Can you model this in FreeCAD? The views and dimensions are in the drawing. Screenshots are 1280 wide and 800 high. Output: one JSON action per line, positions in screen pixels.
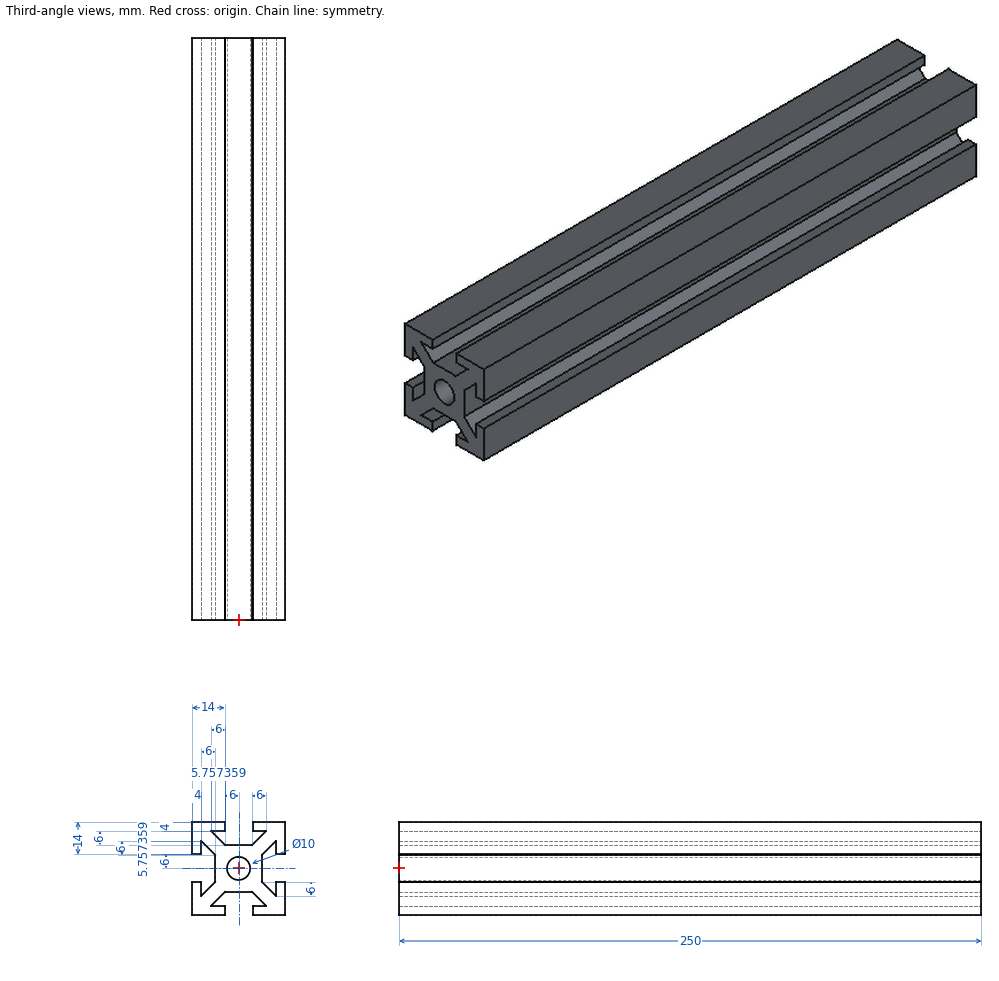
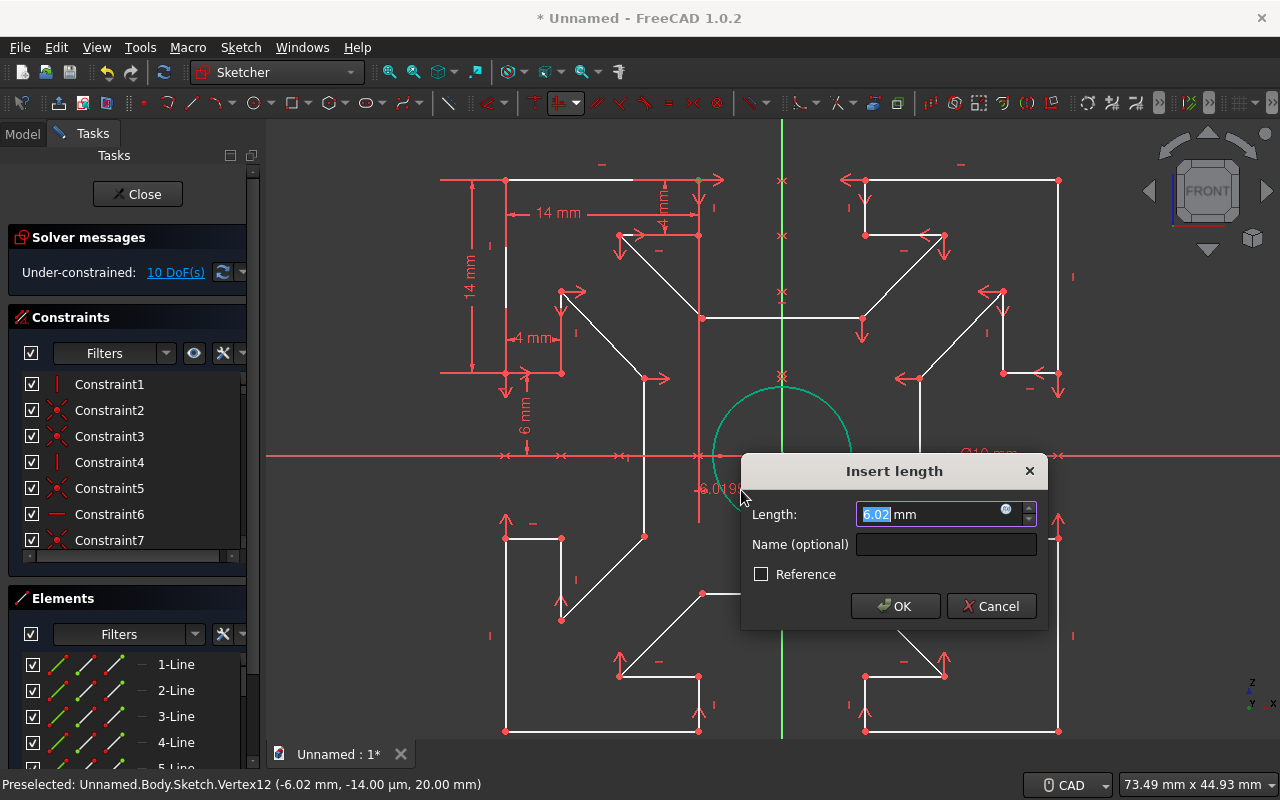
{"action": "type", "text": "6"}
{"action": "key", "text": "Return"}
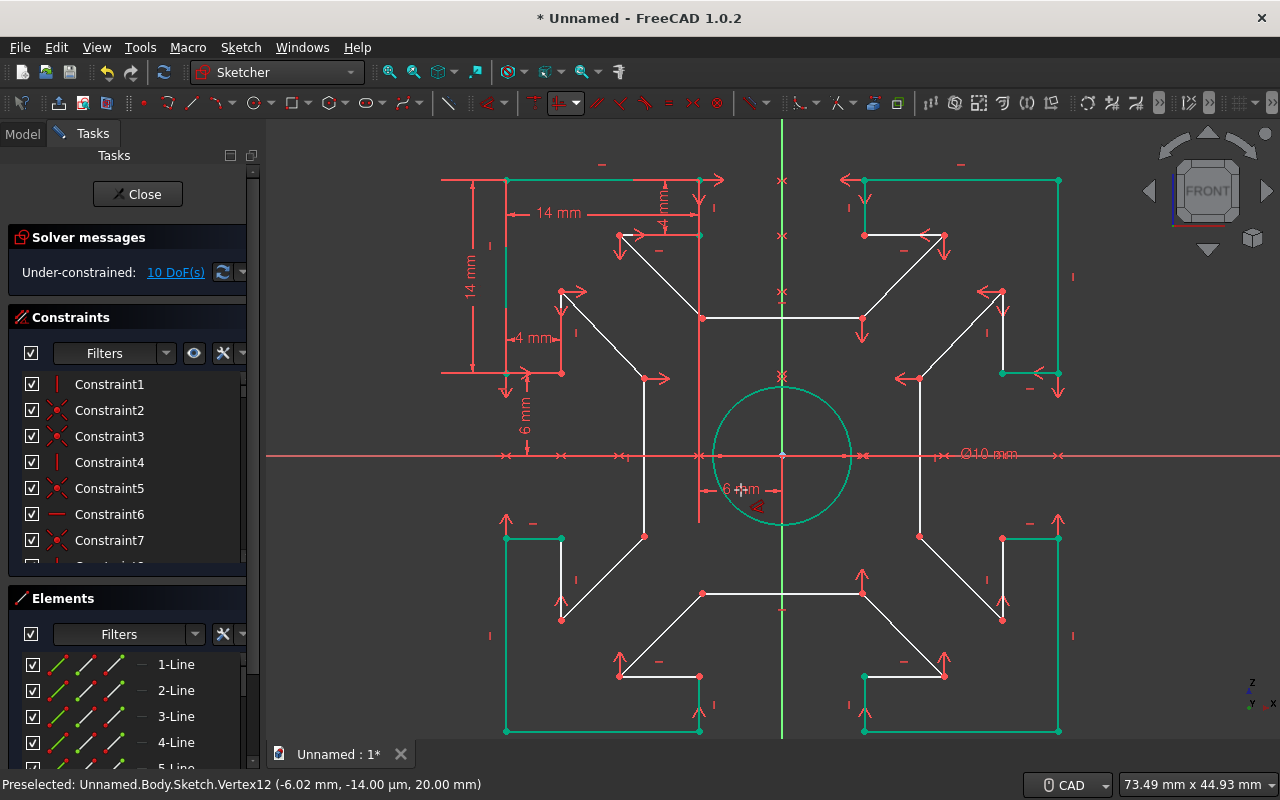
{"action": "left_click", "coordinate": [619, 353]}
{"action": "left_click", "coordinate": [603, 258]}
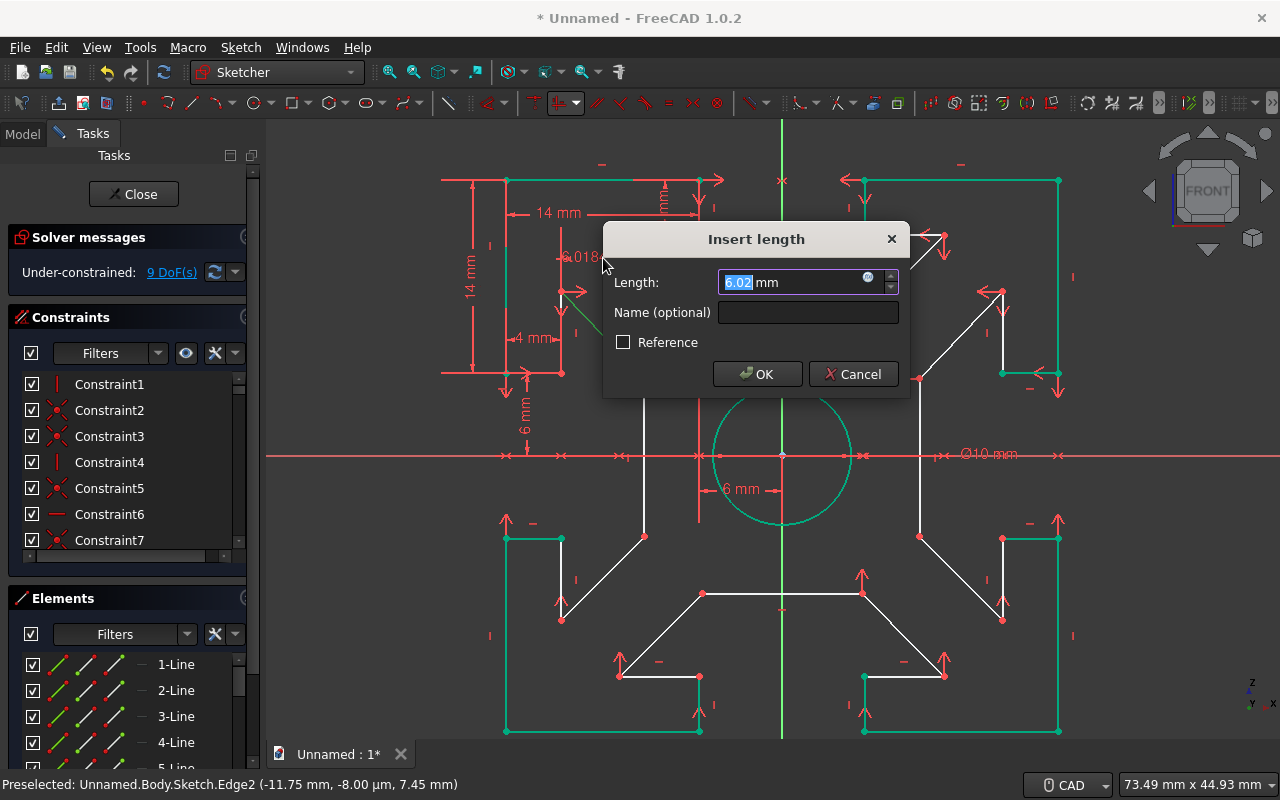
{"action": "type", "text": "6"}
{"action": "key", "text": "Return"}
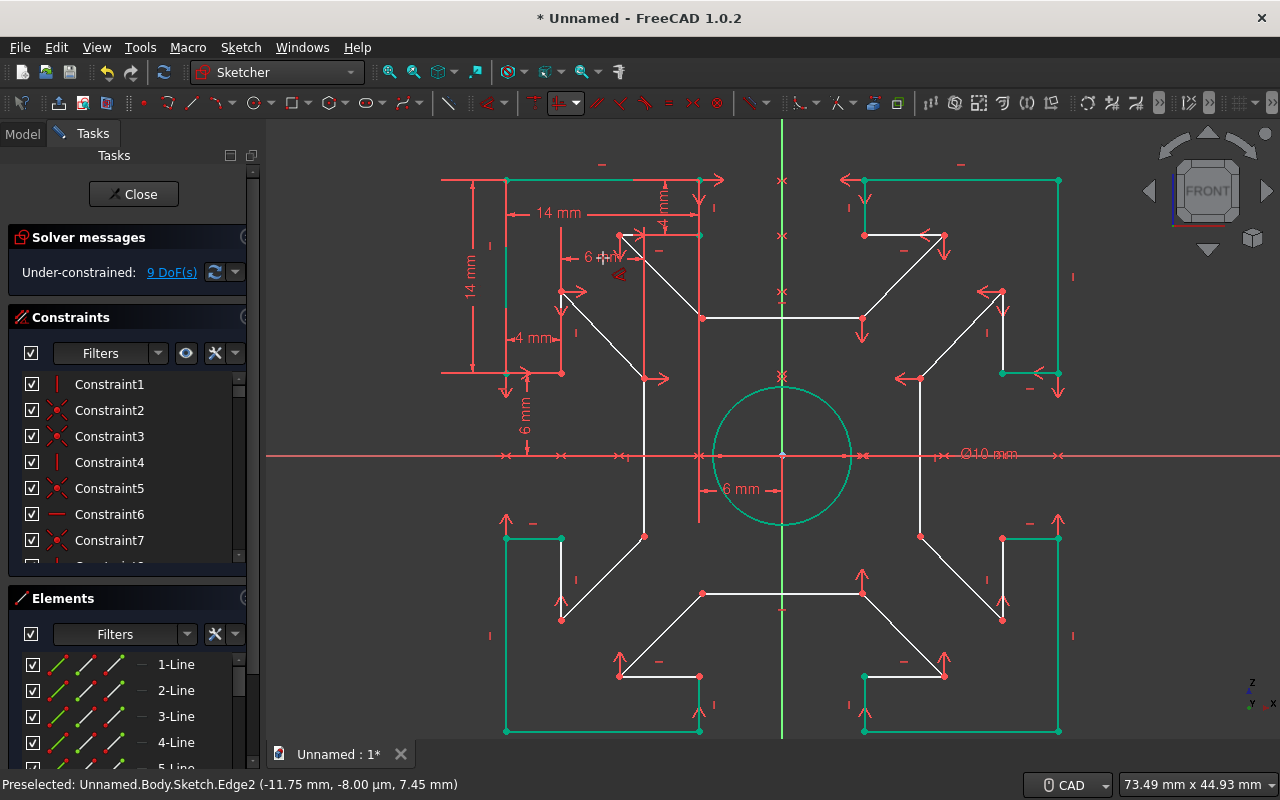
{"action": "left_click", "coordinate": [619, 353]}
{"action": "left_click", "coordinate": [527, 315]}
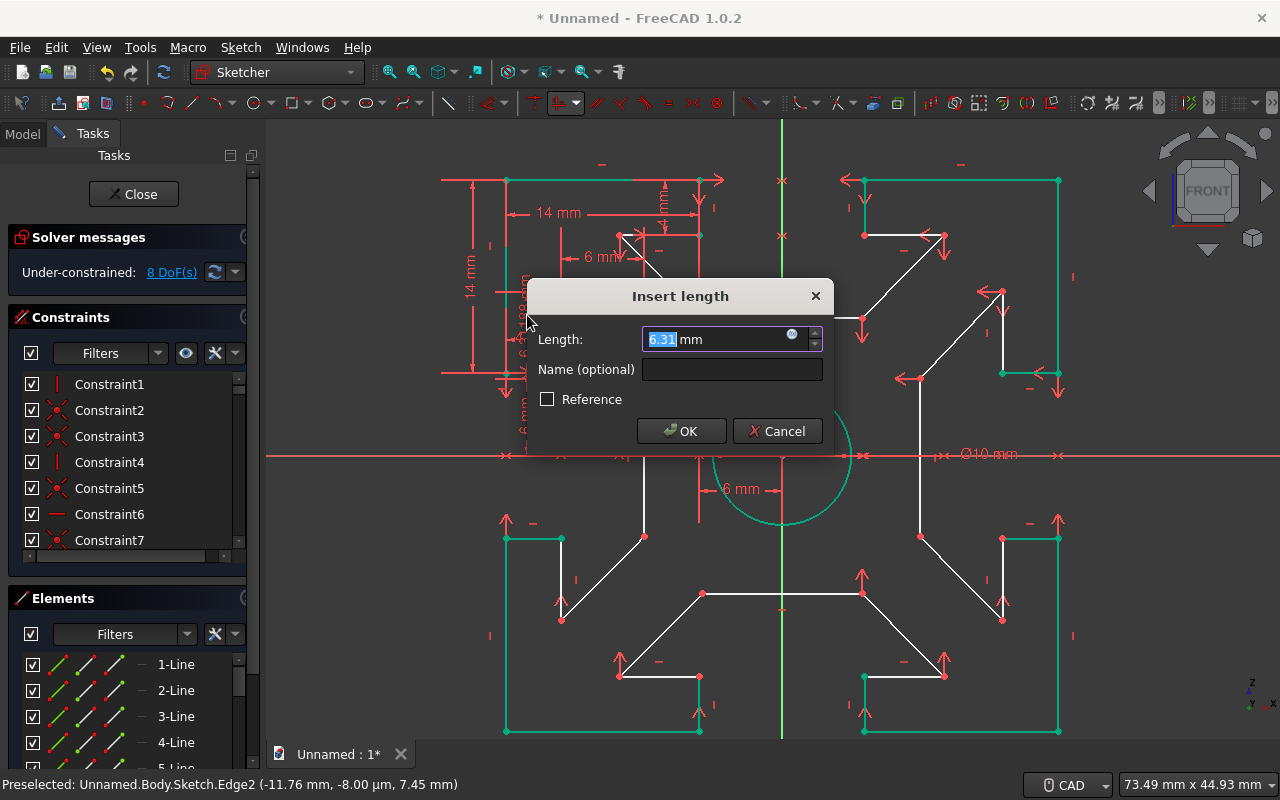
{"action": "type", "text": "6"}
{"action": "key", "text": "Return"}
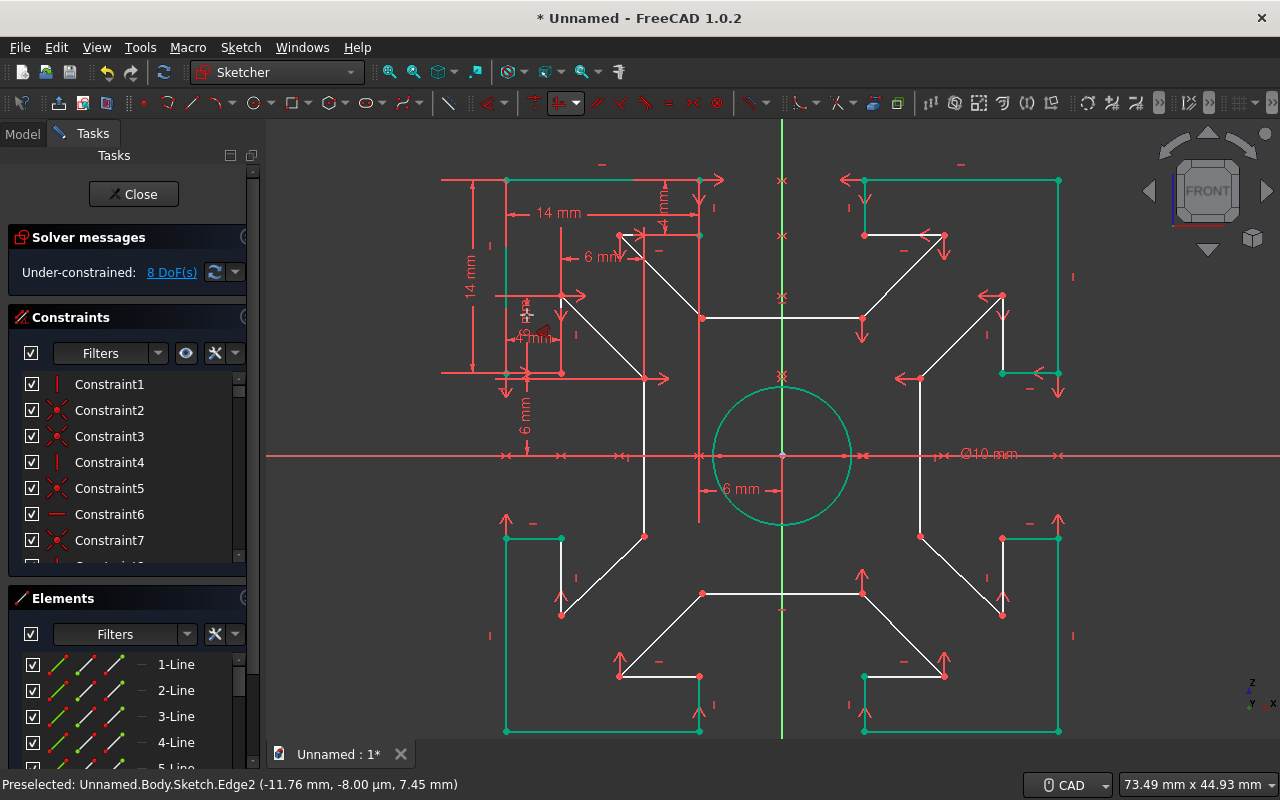
{"action": "left_click", "coordinate": [645, 260]}
{"action": "left_click", "coordinate": [661, 352]}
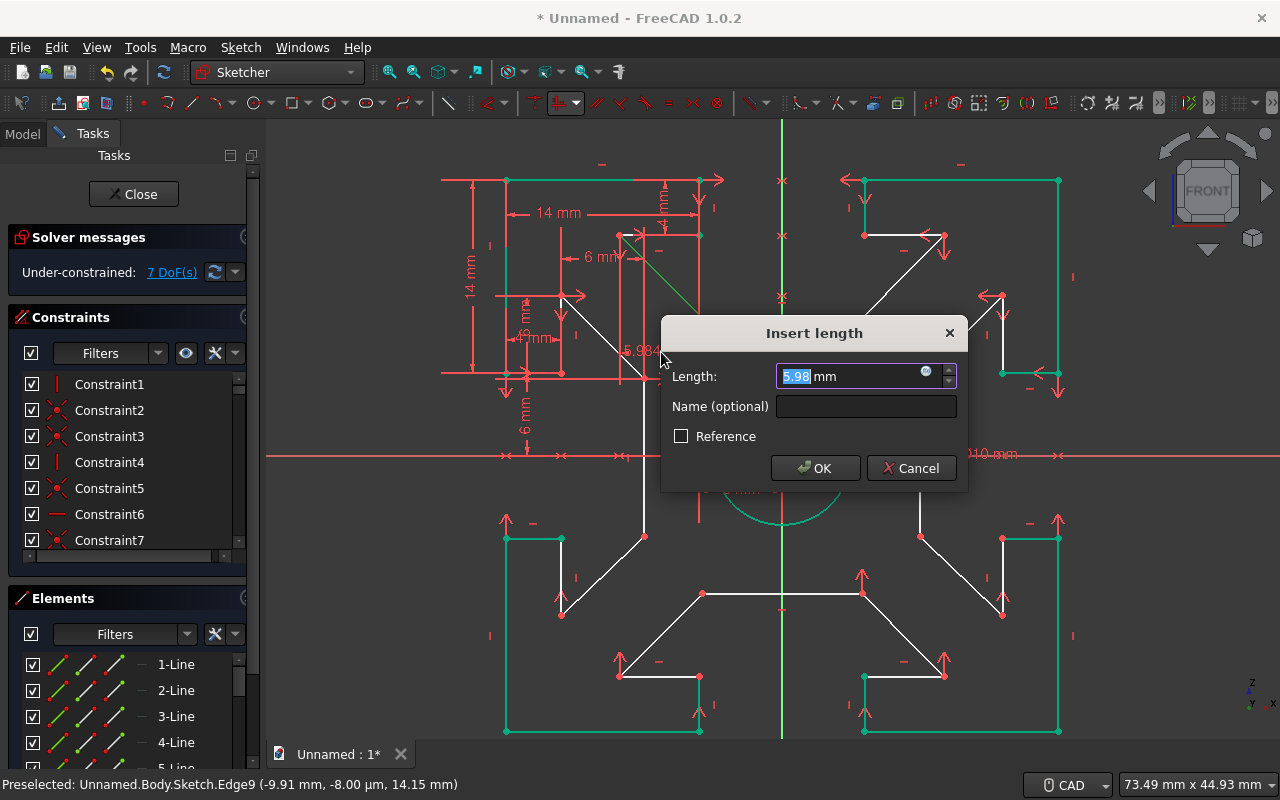
{"action": "type", "text": "6"}
{"action": "key", "text": "Return"}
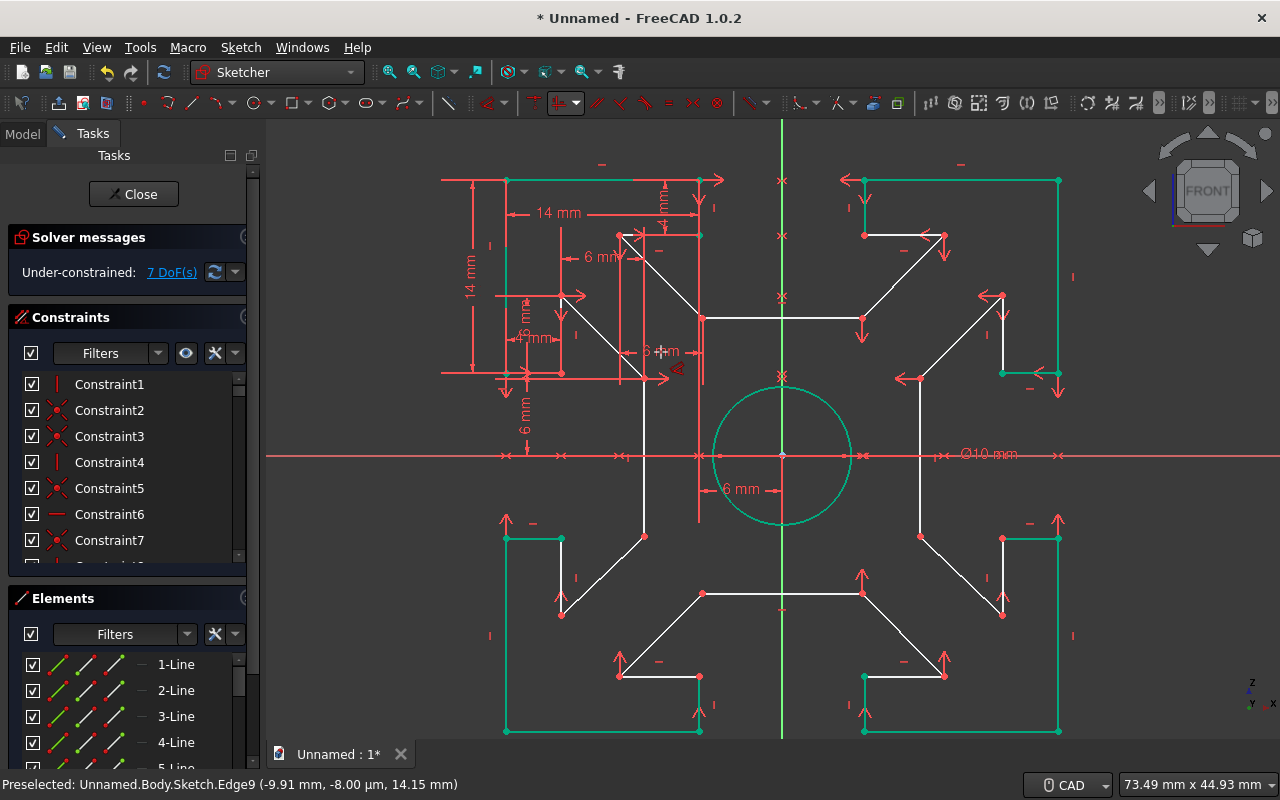
{"action": "left_click", "coordinate": [645, 260]}
{"action": "left_click", "coordinate": [737, 277]}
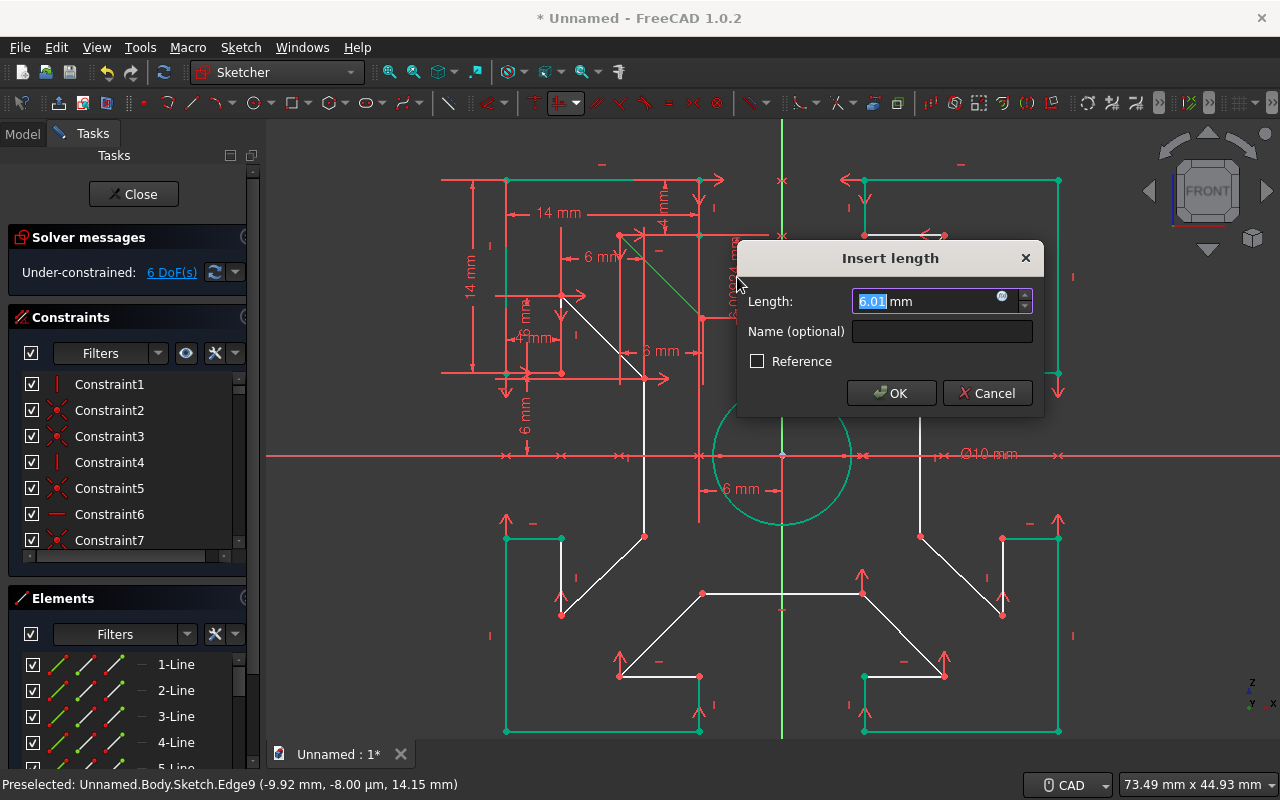
{"action": "type", "text": "6"}
{"action": "key", "text": "Return"}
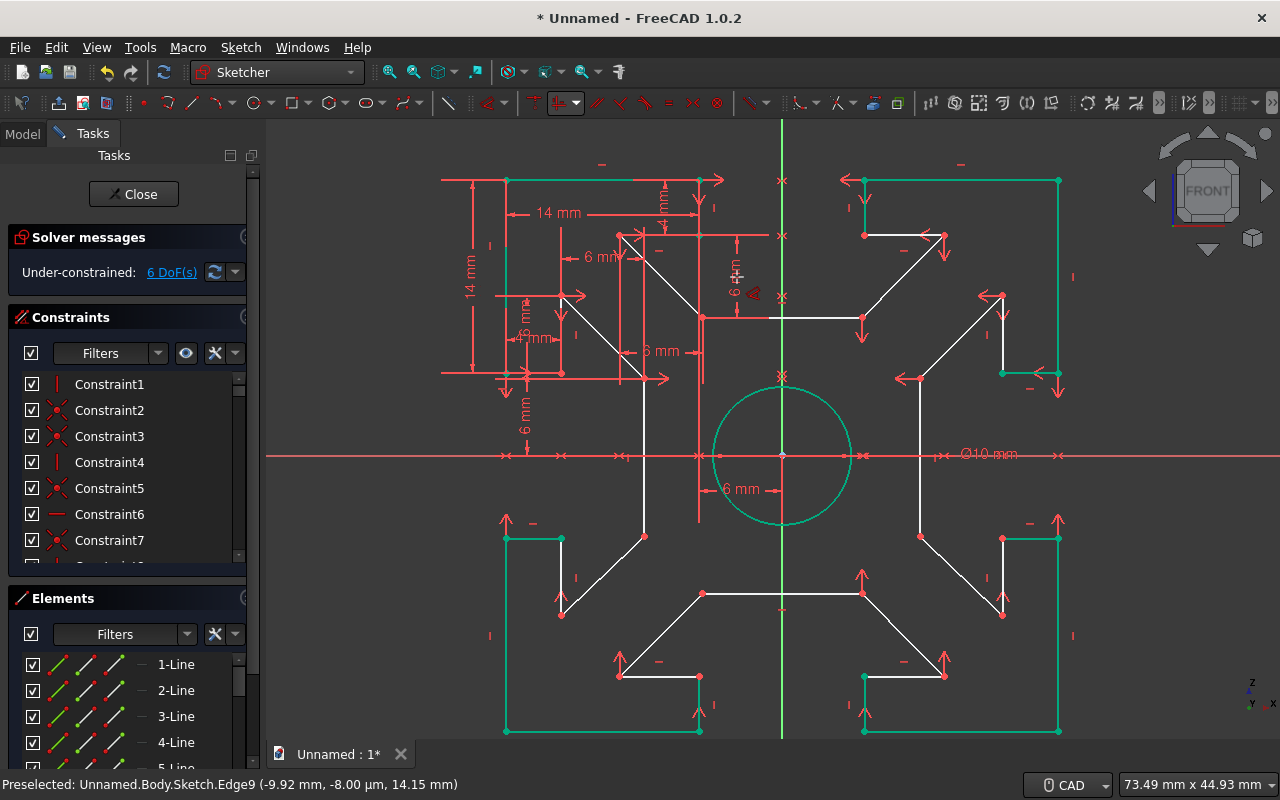
{"action": "left_click", "coordinate": [887, 293]}
{"action": "left_click", "coordinate": [903, 201]}